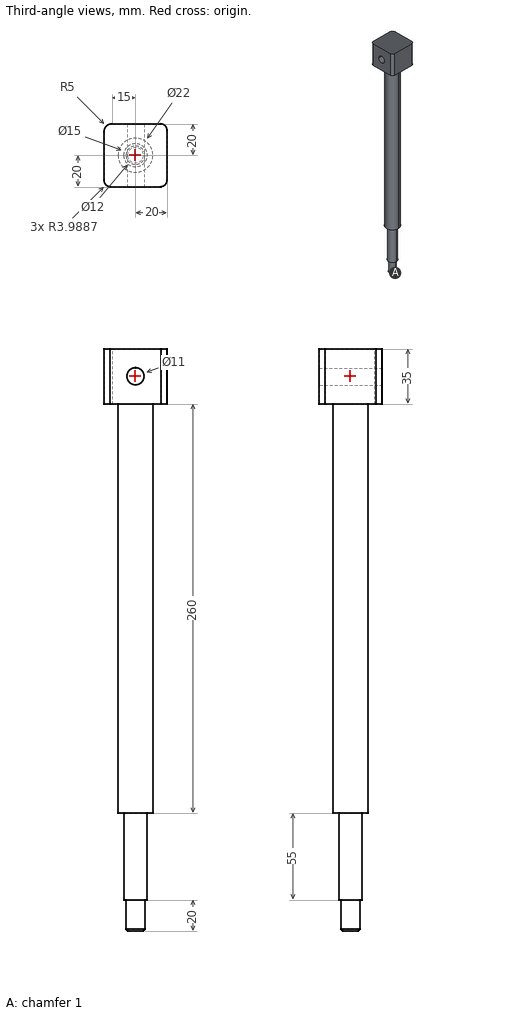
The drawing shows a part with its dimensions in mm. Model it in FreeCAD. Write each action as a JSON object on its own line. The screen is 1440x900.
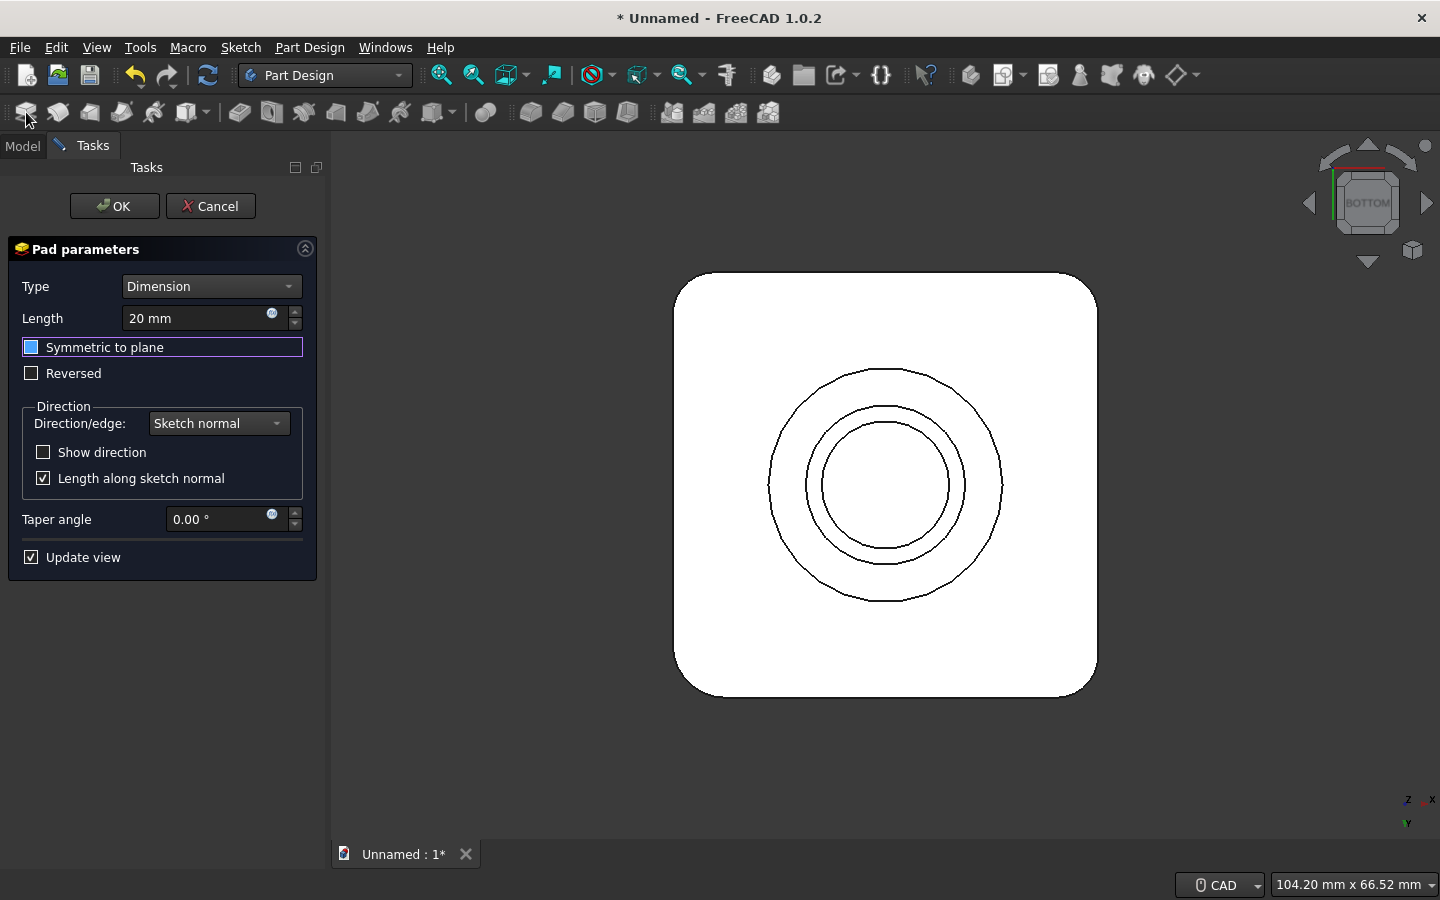
{"action": "left_click", "coordinate": [115, 206]}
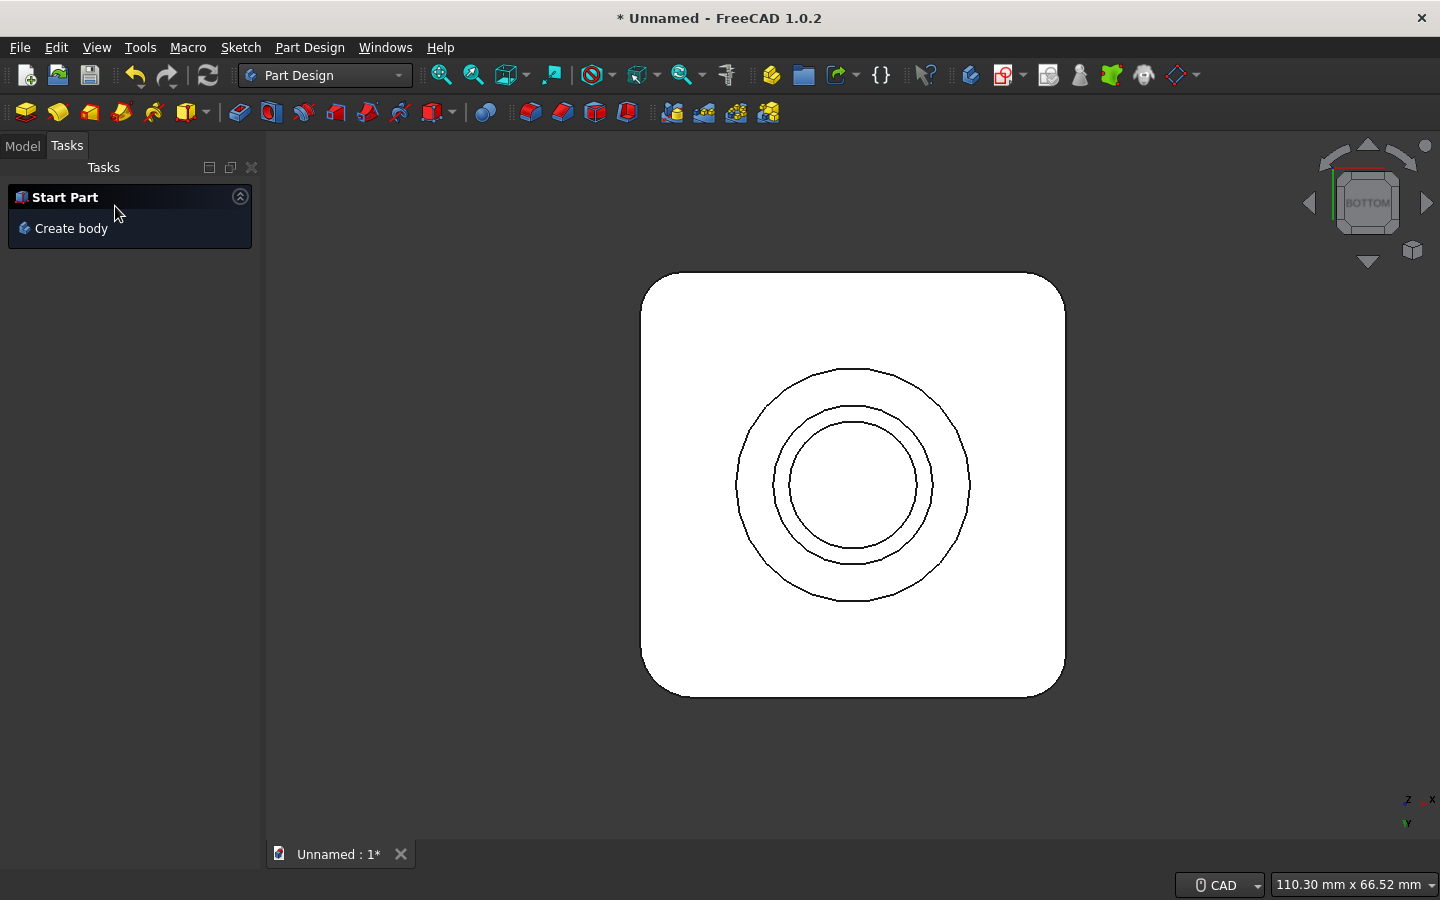
{"action": "left_click", "coordinate": [789, 484]}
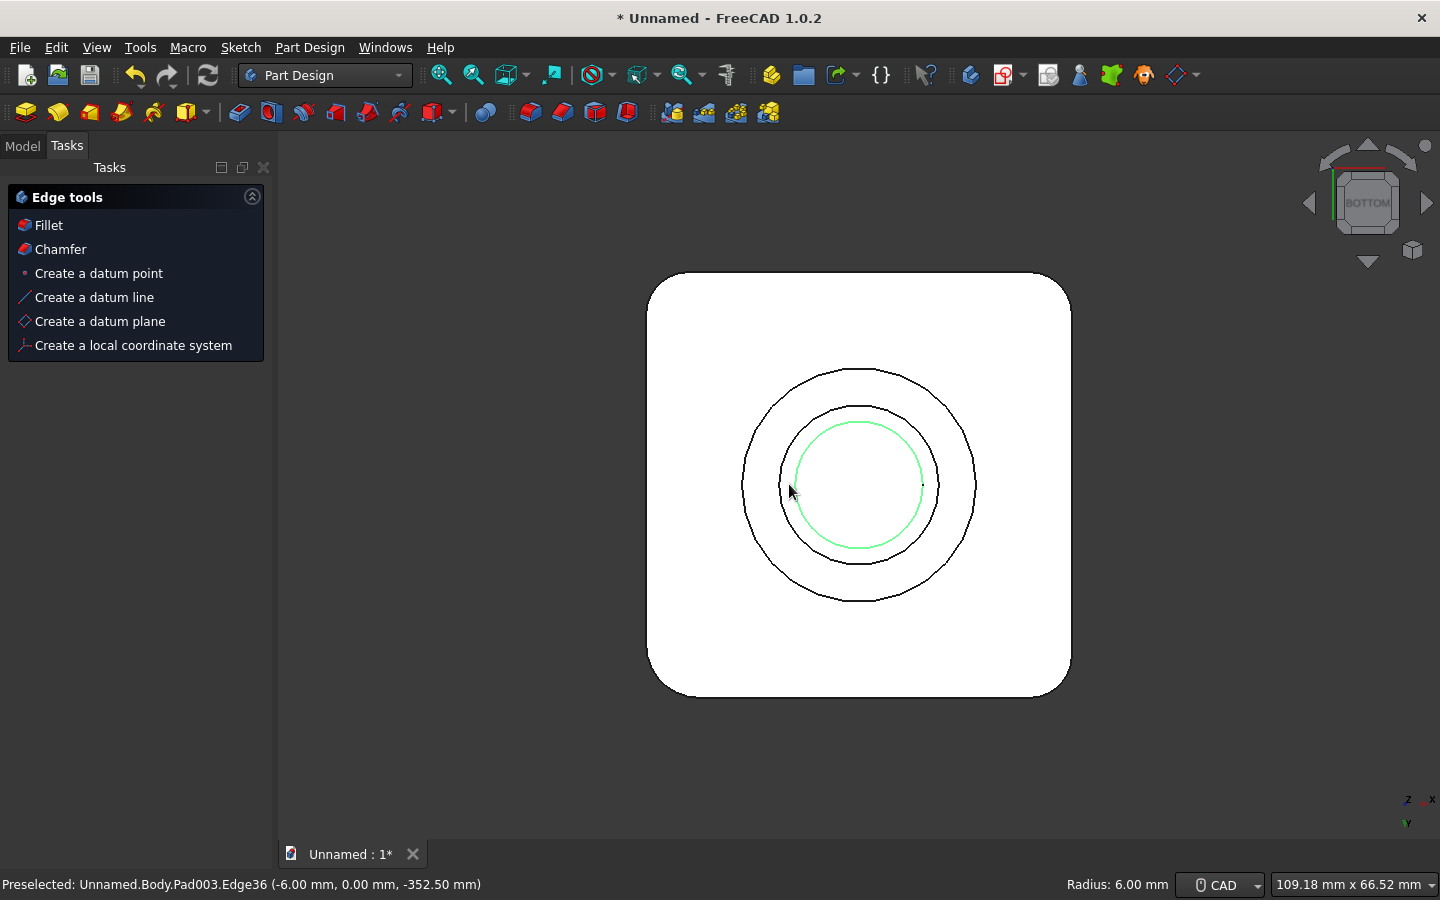
{"action": "left_click", "coordinate": [564, 112]}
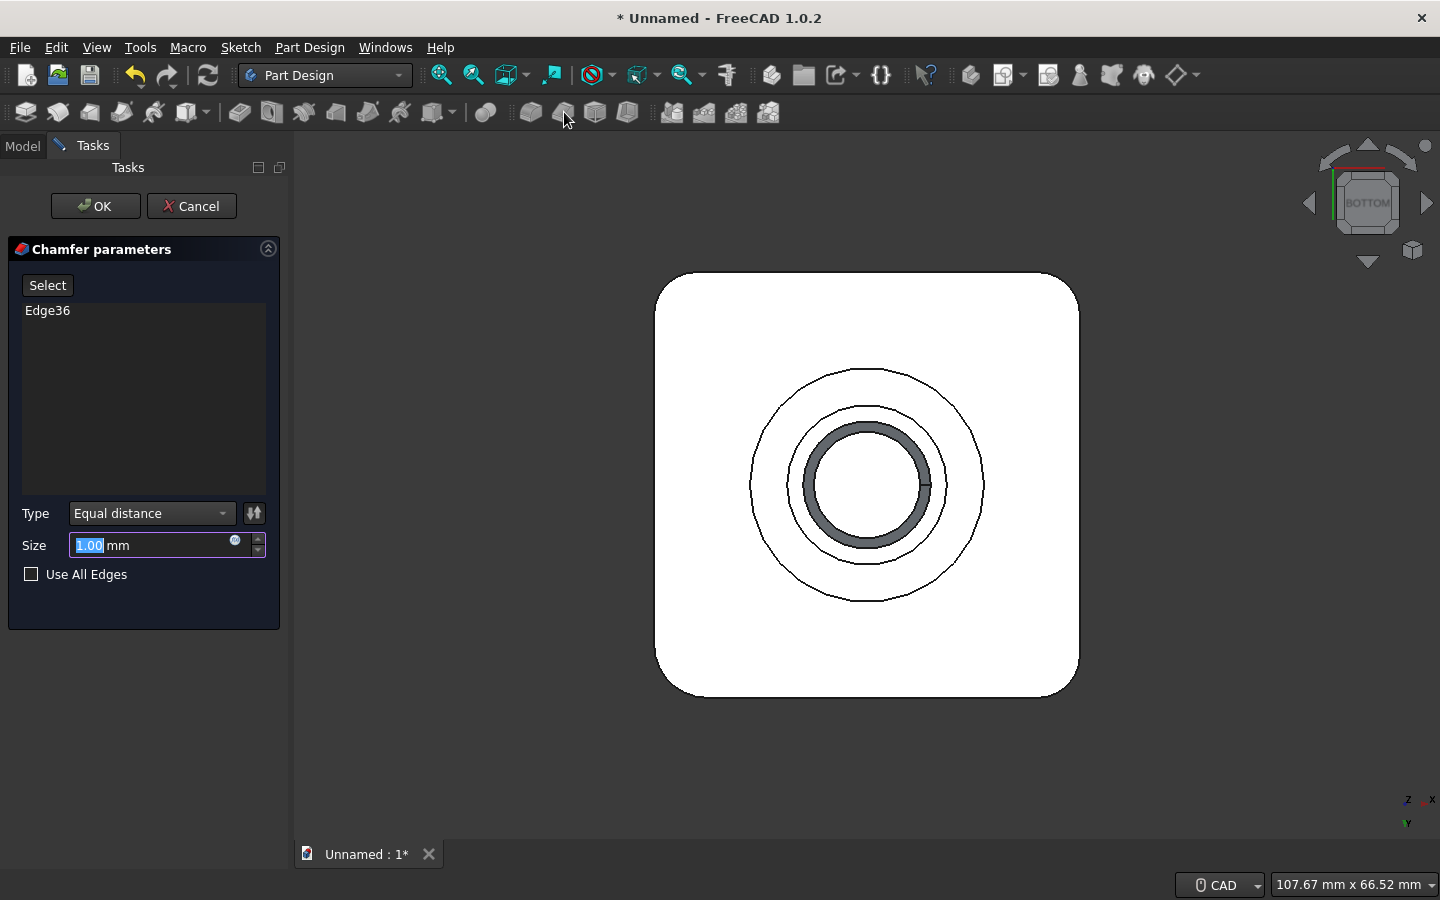
{"action": "type", "text": "1"}
{"action": "key", "text": "Tab"}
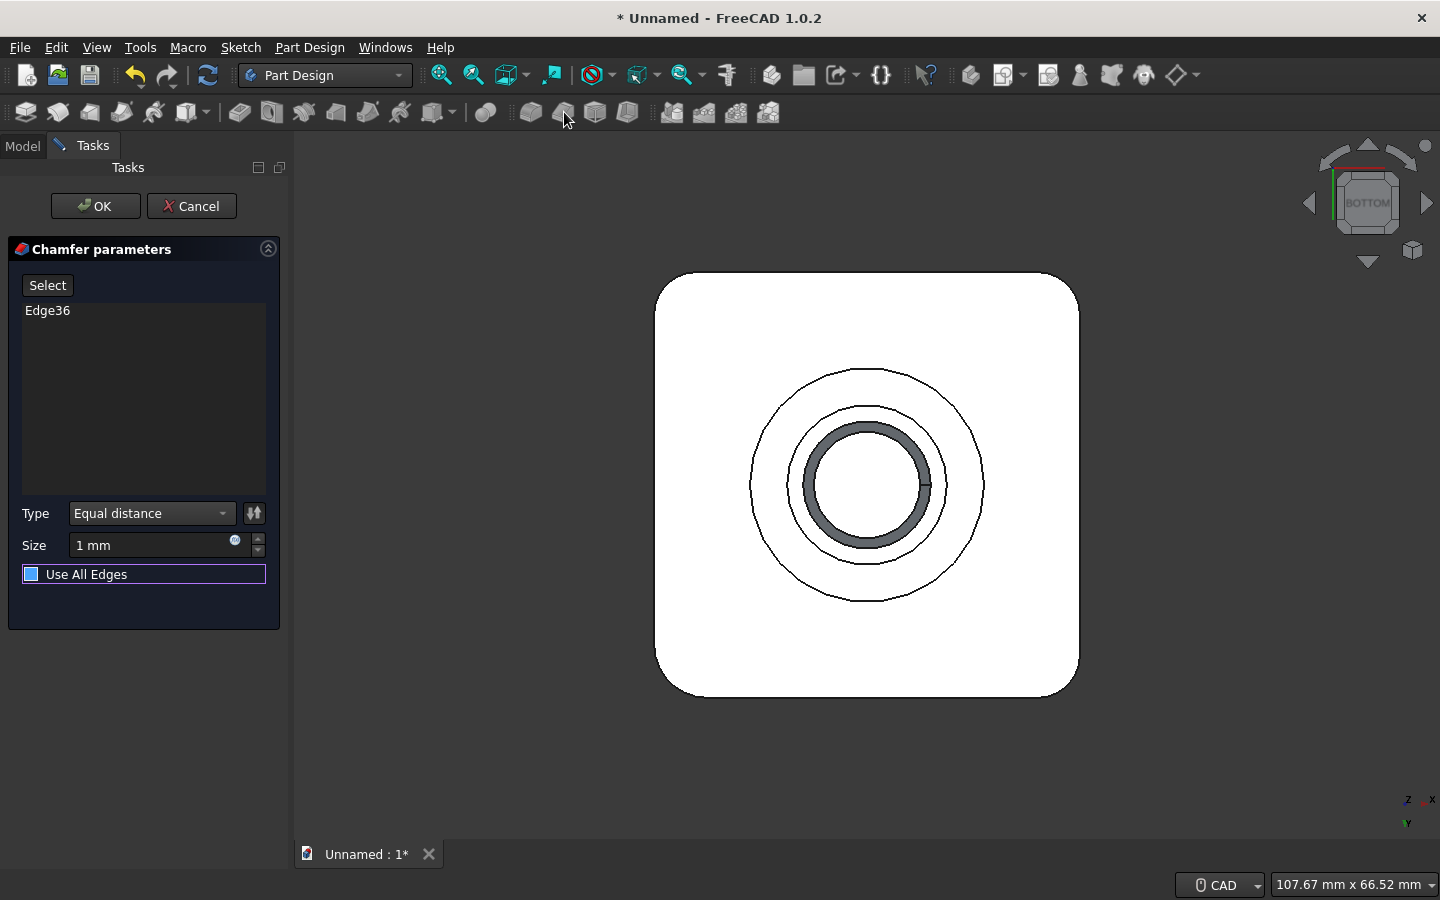
{"action": "left_click", "coordinate": [96, 206]}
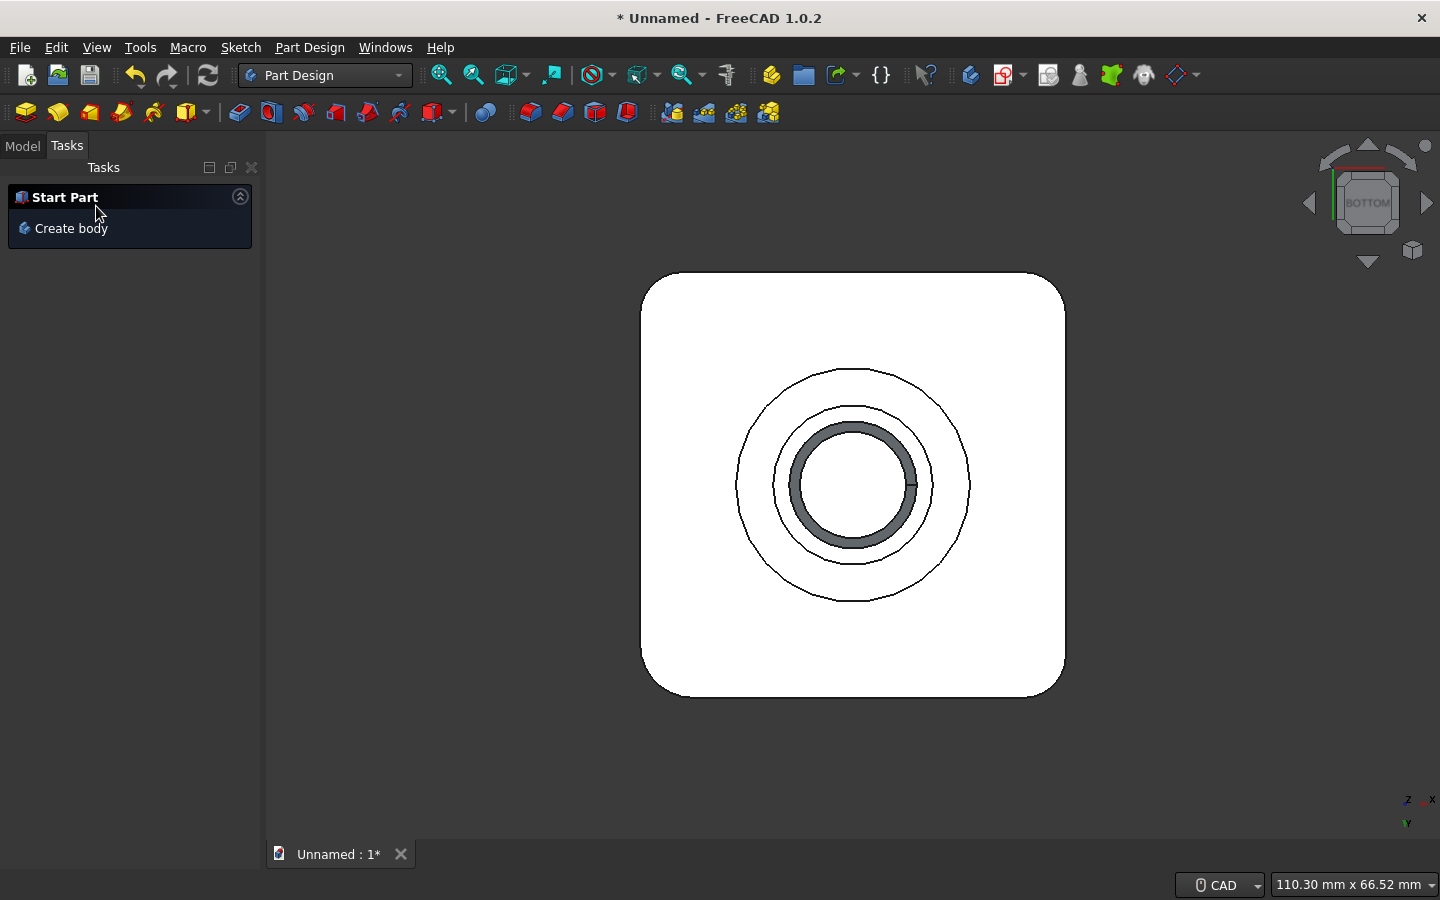
{"action": "key", "text": "0"}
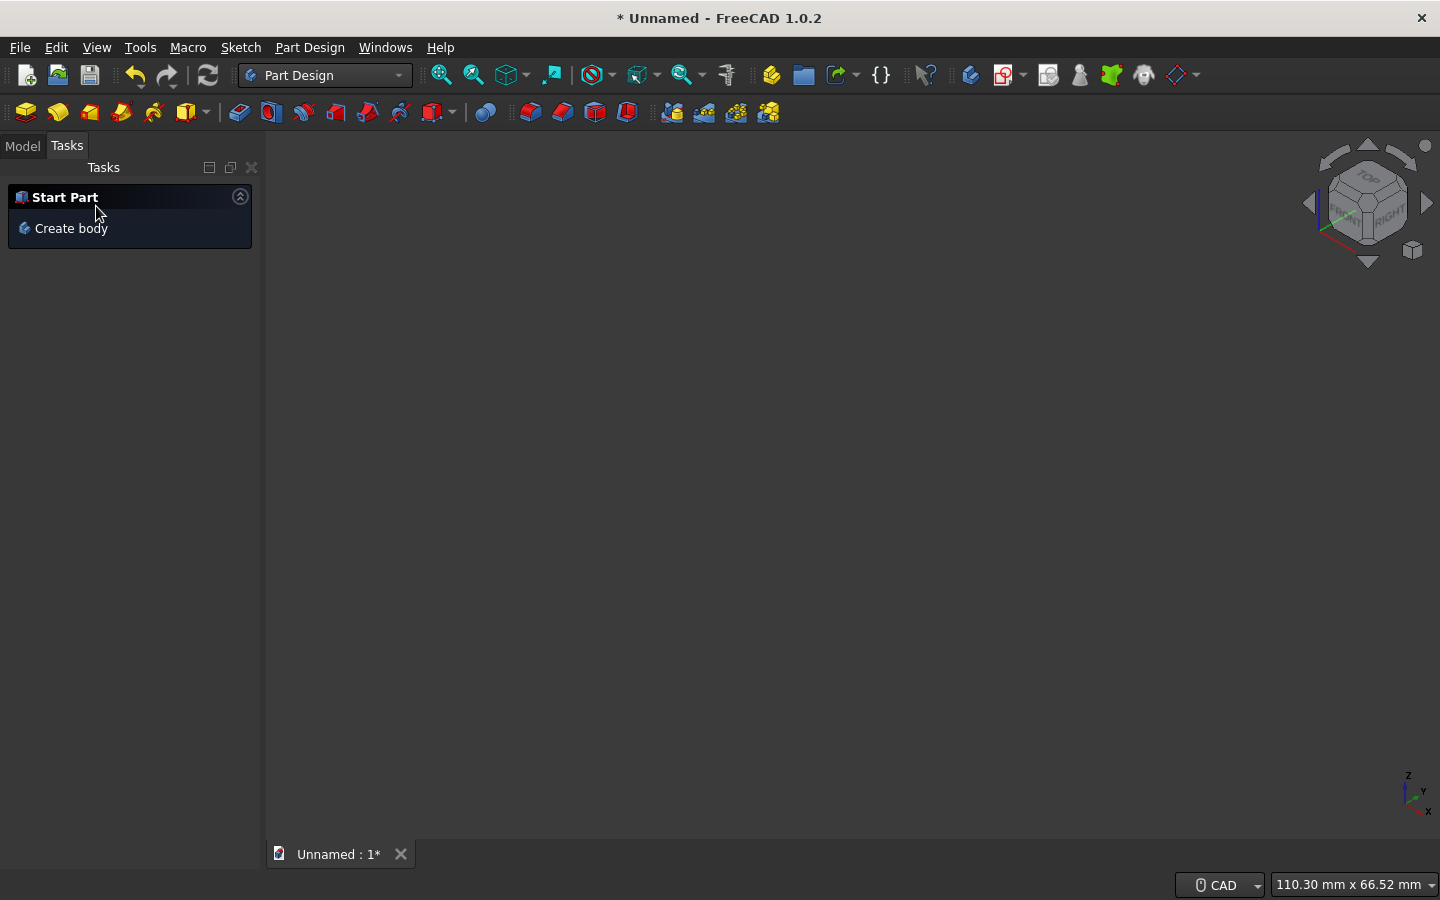
{"action": "left_click", "coordinate": [442, 76]}